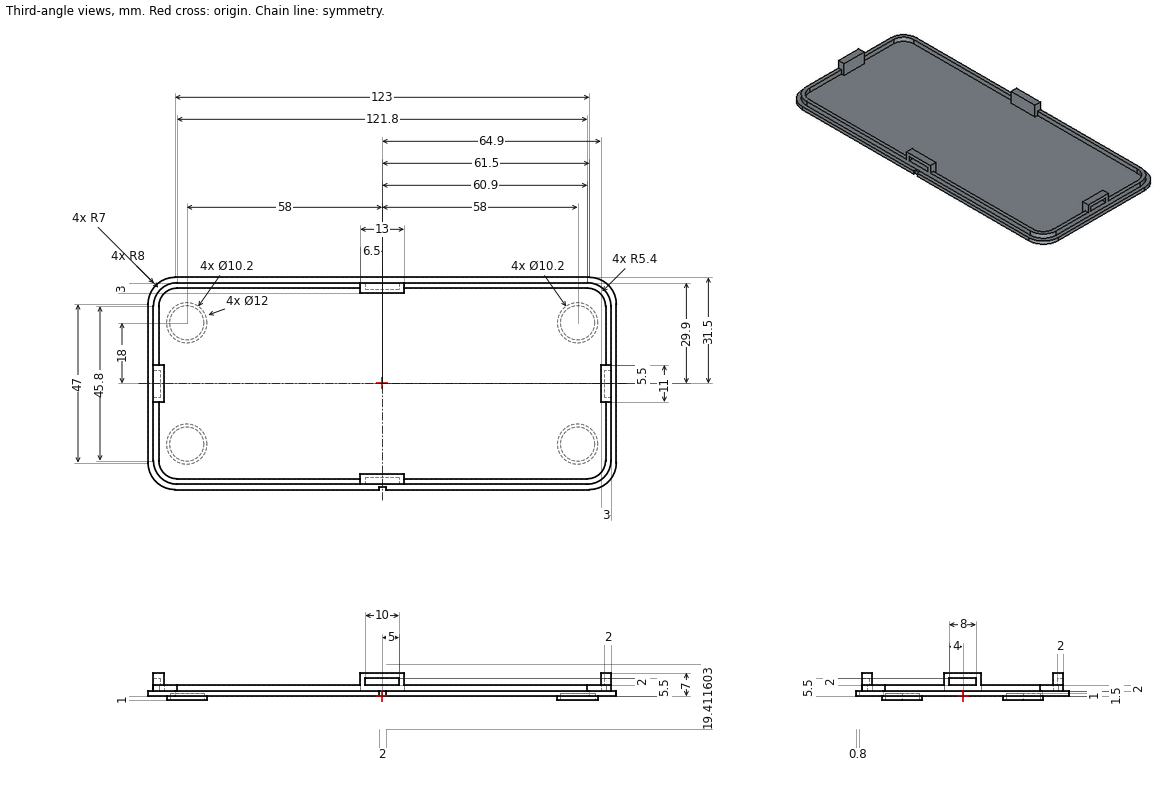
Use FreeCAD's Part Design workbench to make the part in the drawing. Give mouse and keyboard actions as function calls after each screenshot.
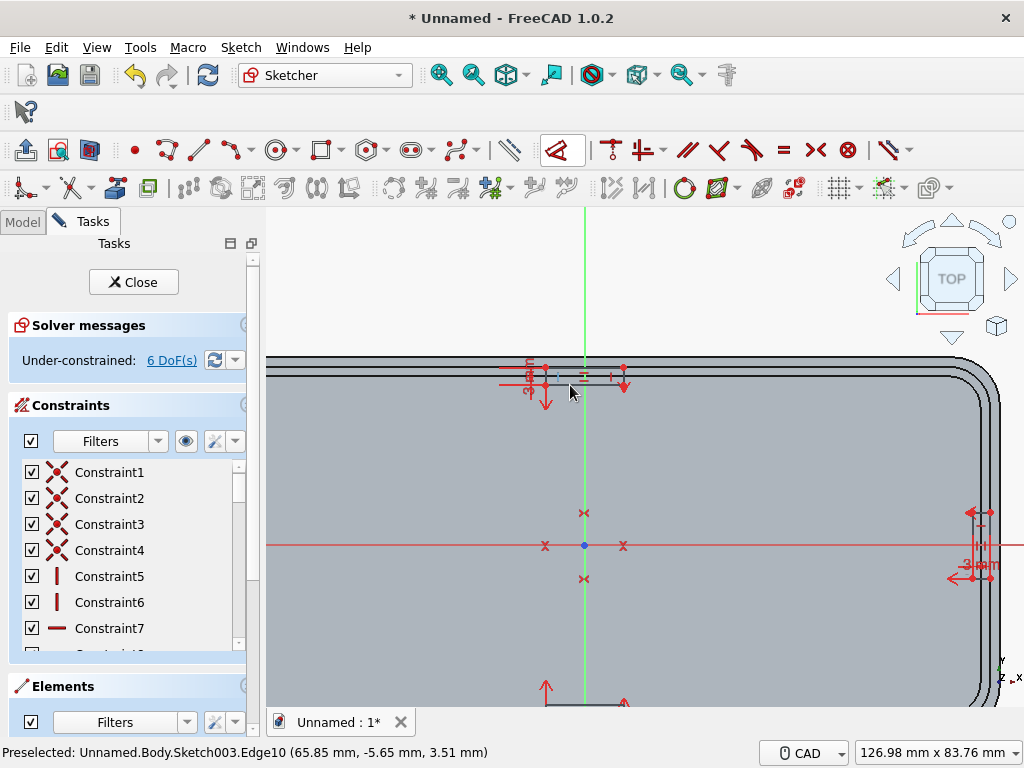
click(569, 385)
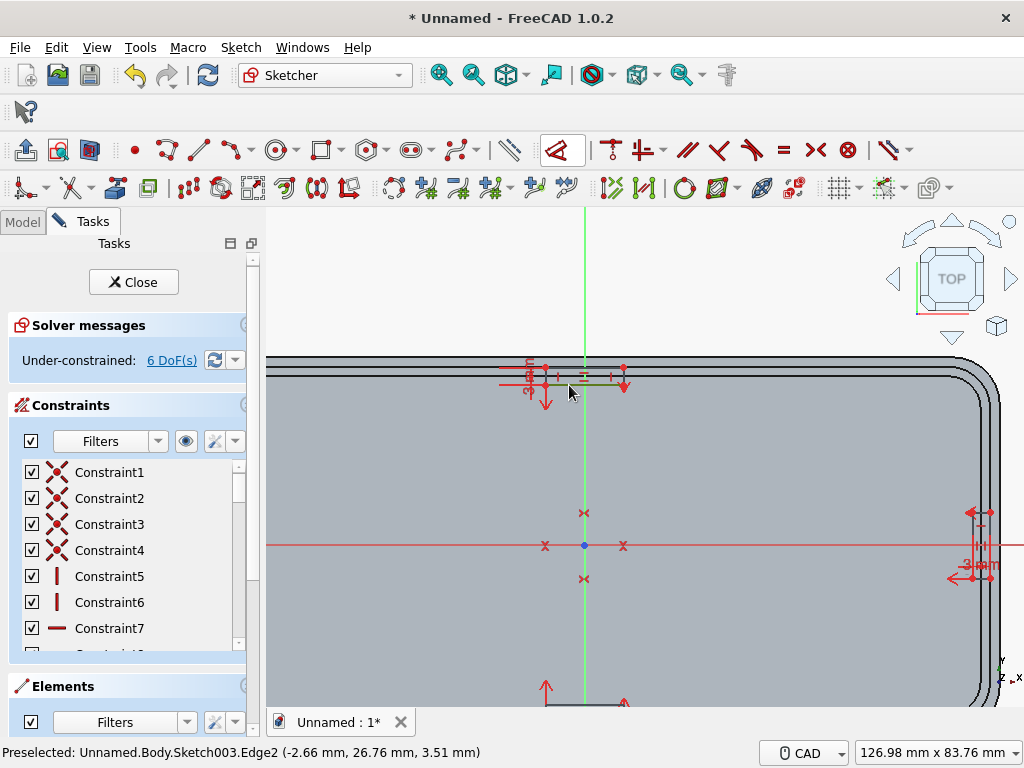
key(l)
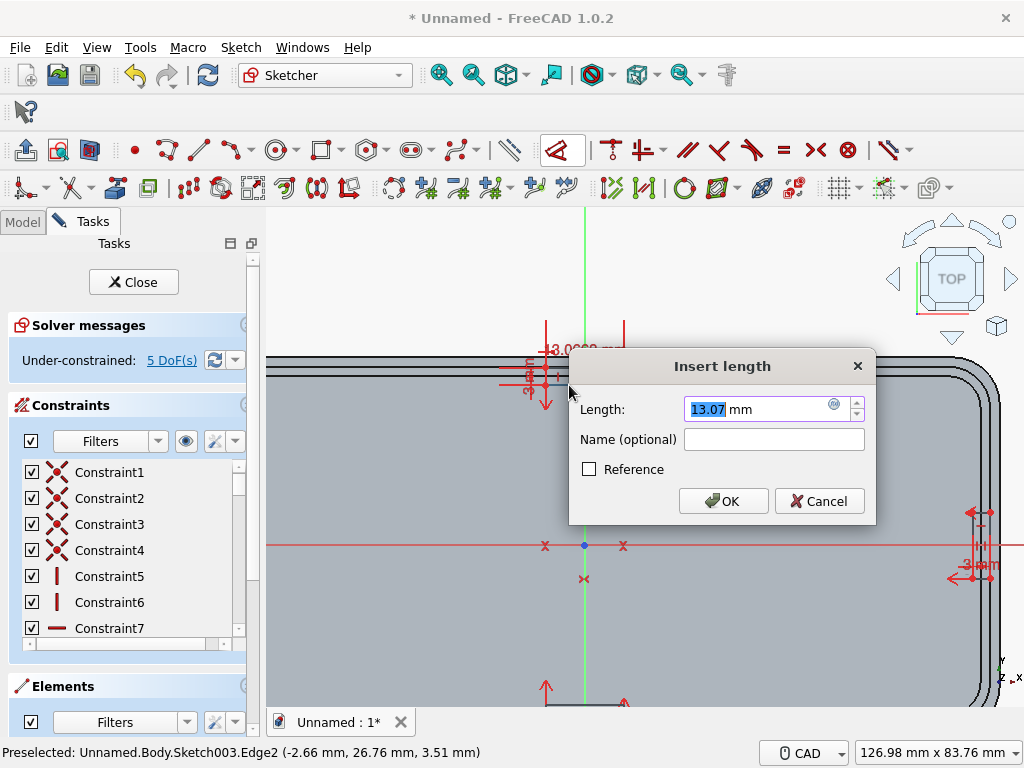
text(13)
key(Return)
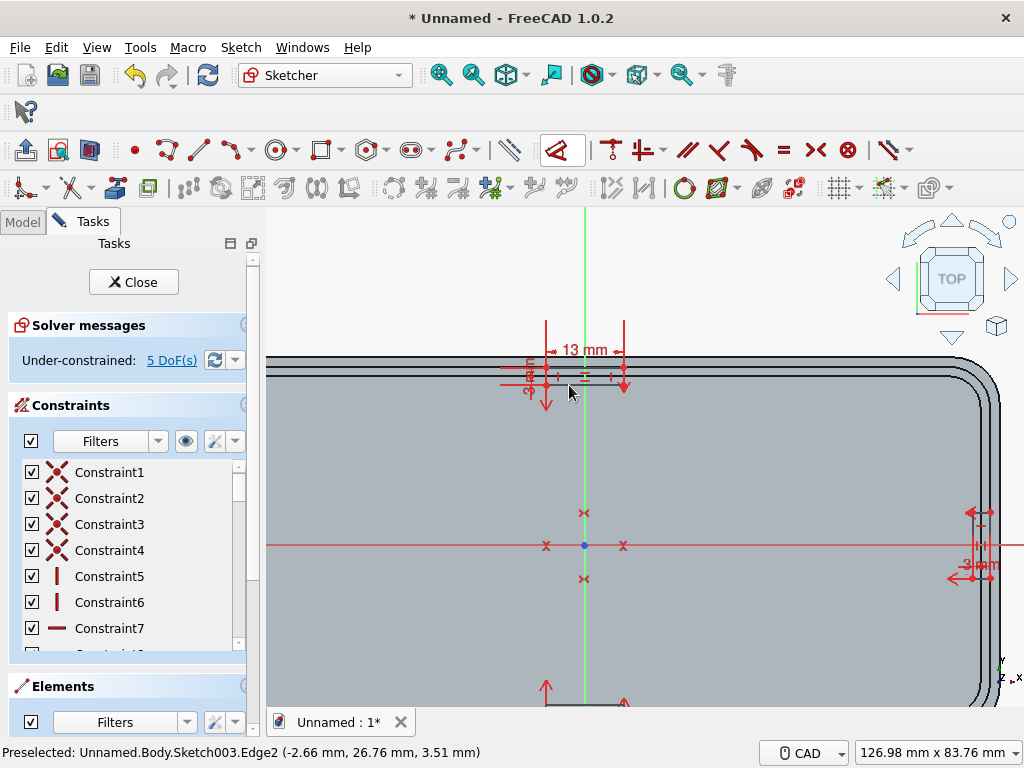
scroll(570, 385, down, 4)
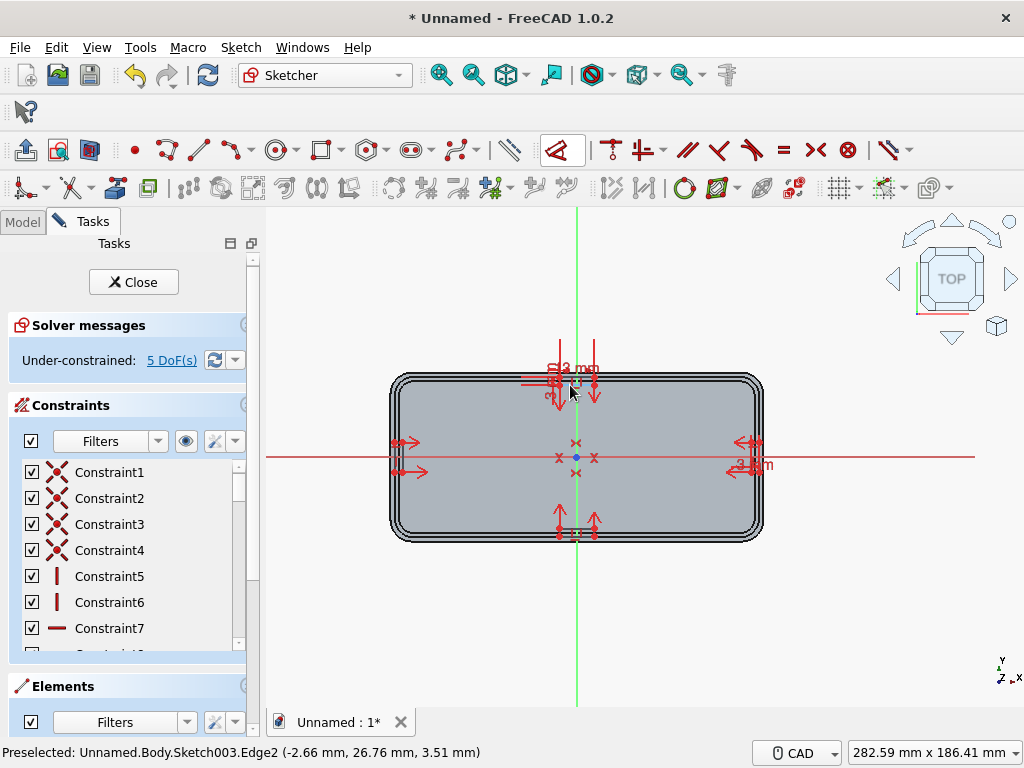
scroll(751, 452, up, 5)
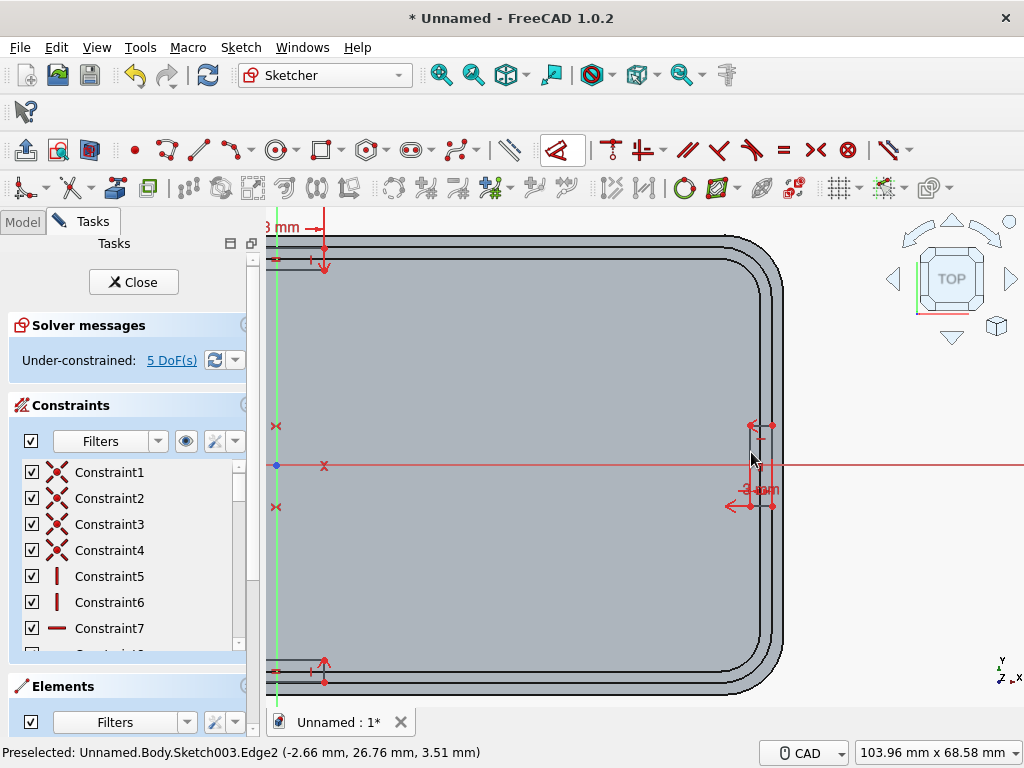
click(750, 450)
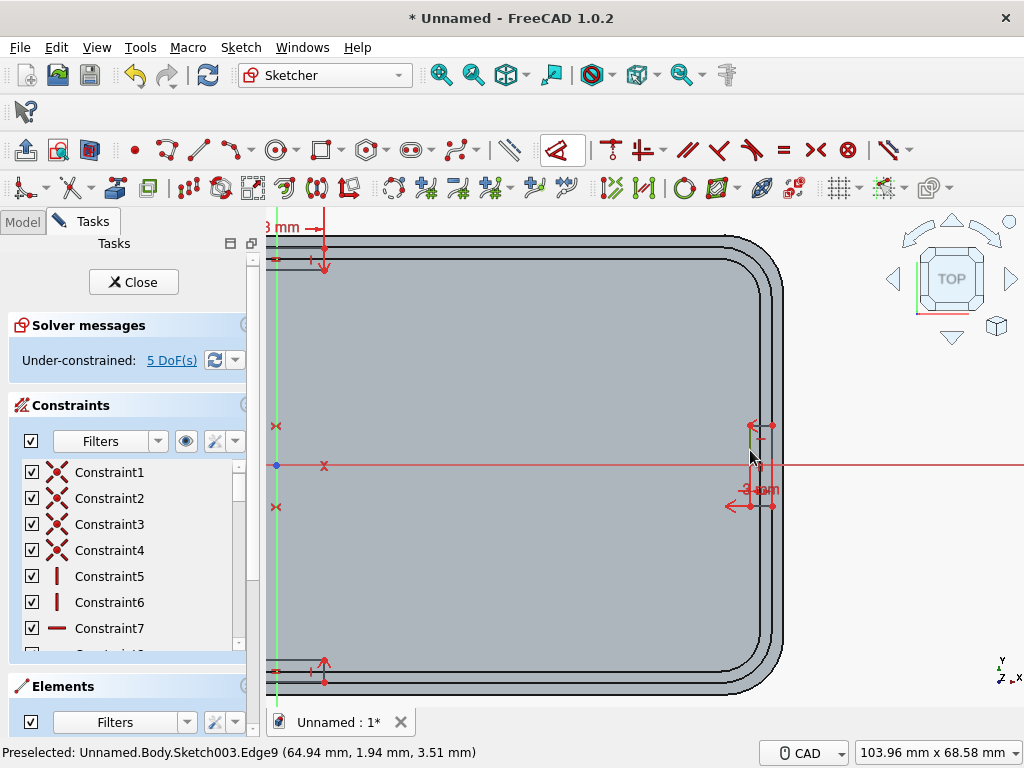
key(i)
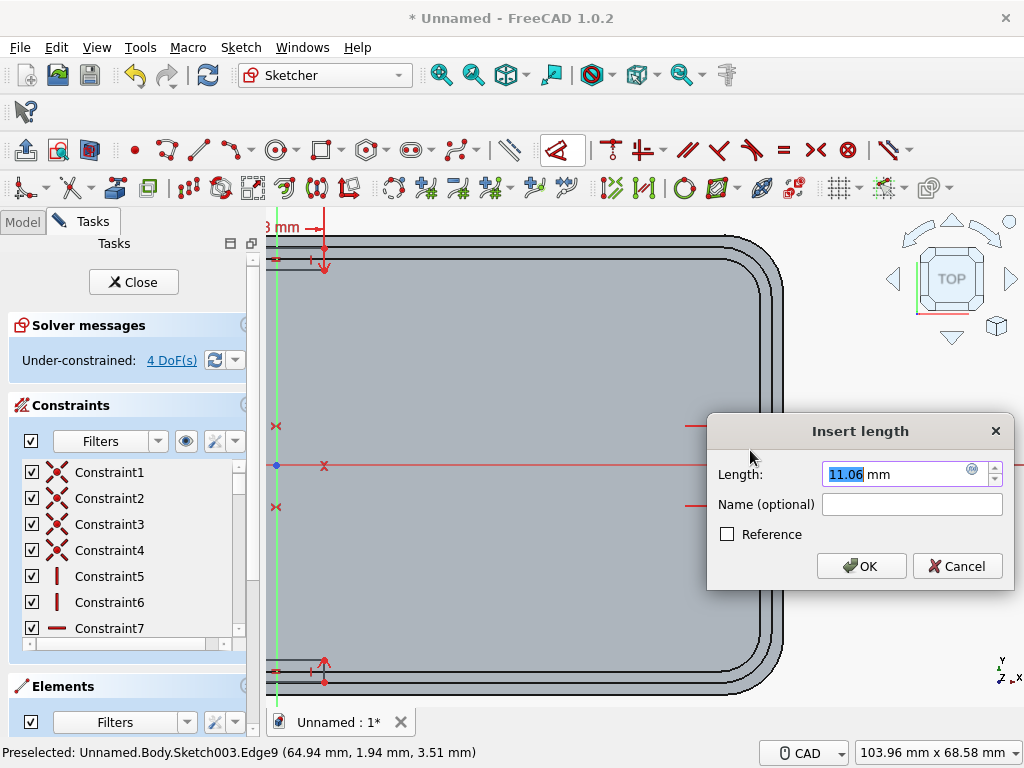
text(11)
key(Return)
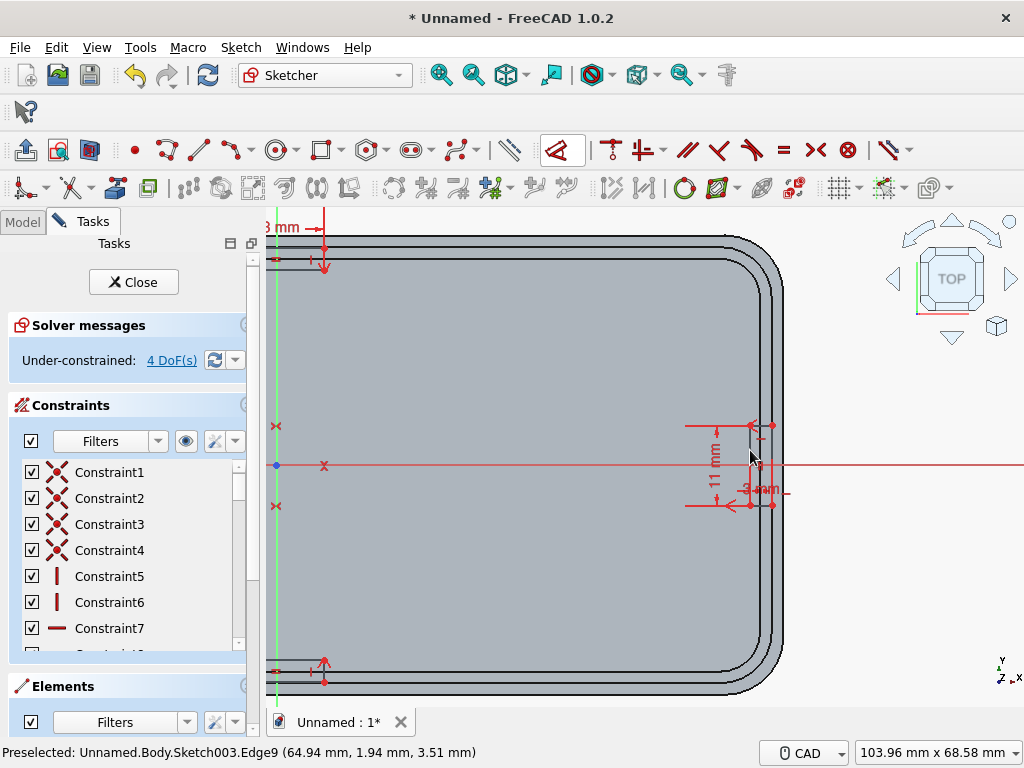
scroll(751, 452, down, 5)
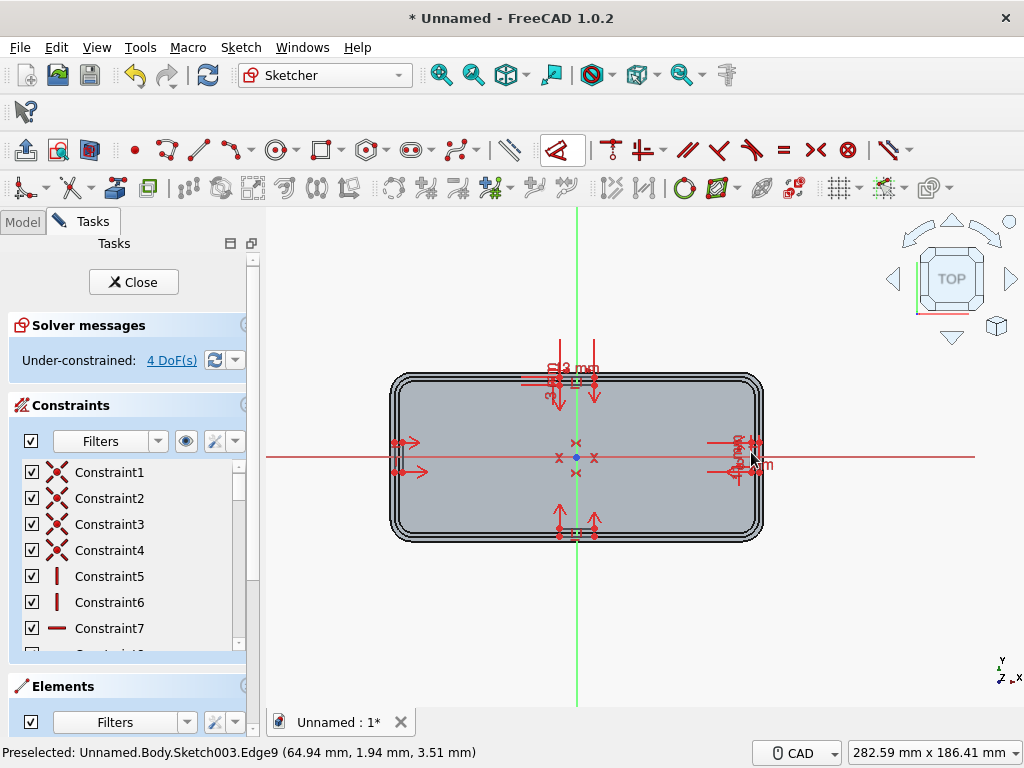
scroll(560, 377, up, 5)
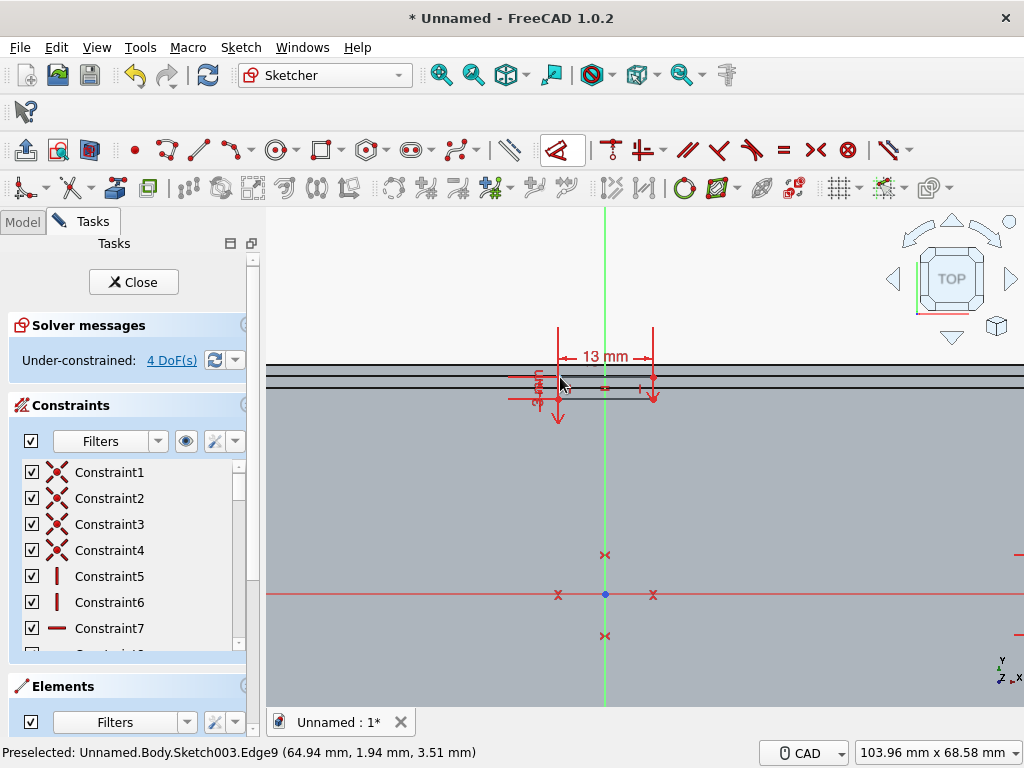
click(558, 377)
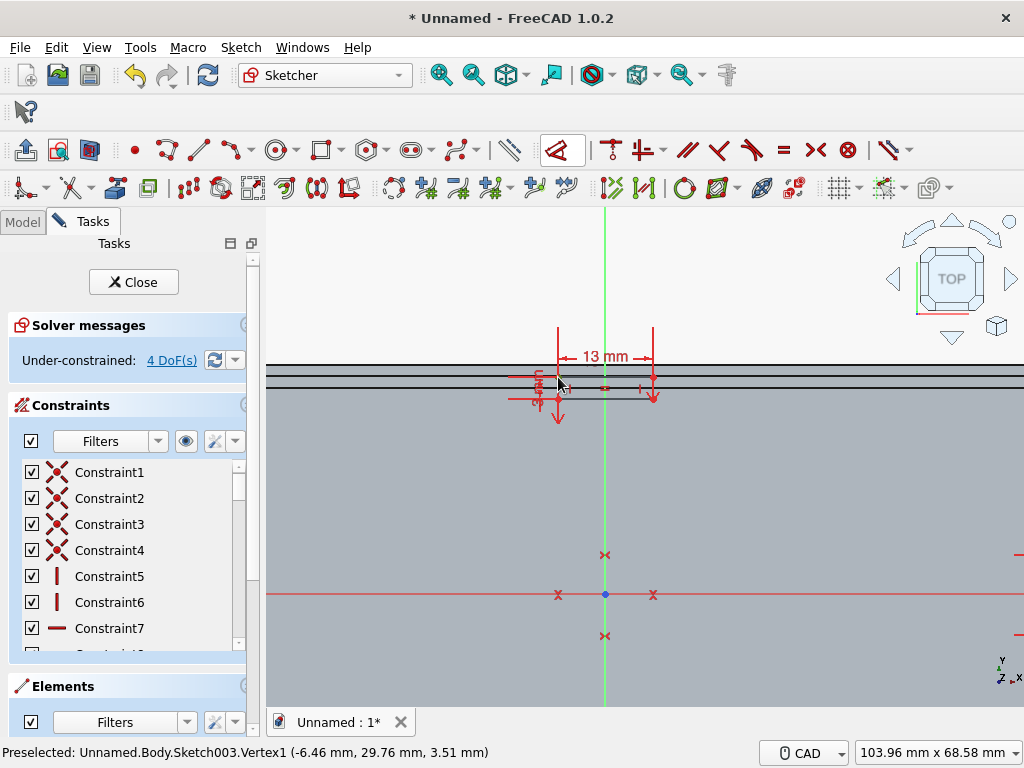
key(l)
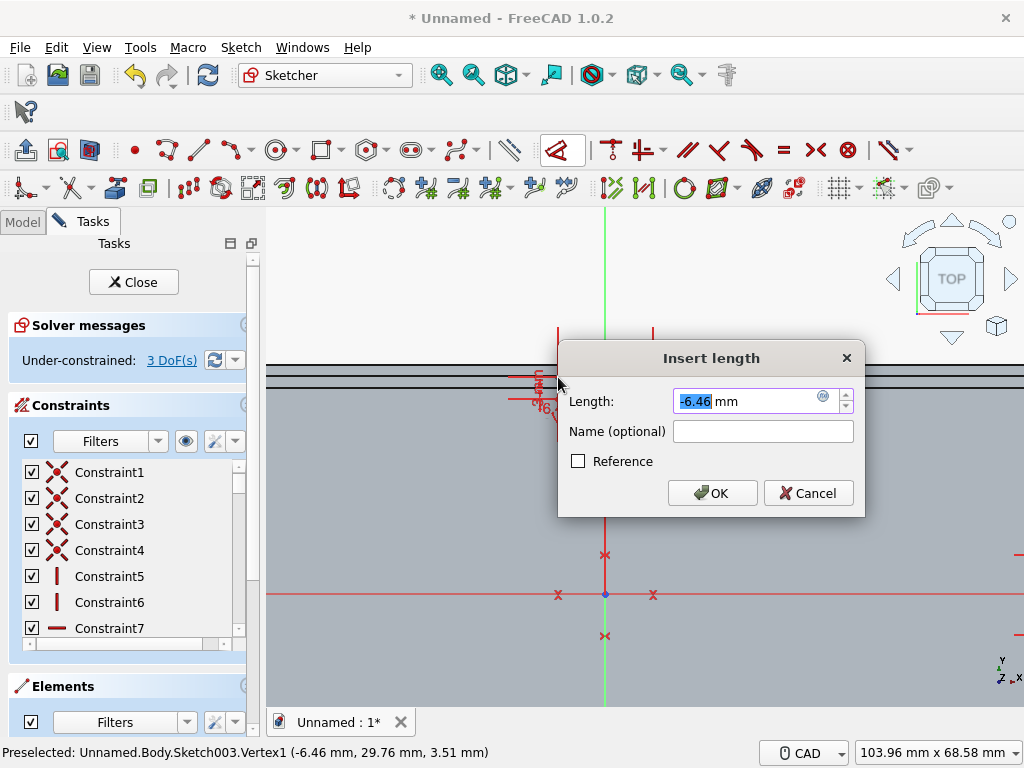
text(-6.5)
key(Return)